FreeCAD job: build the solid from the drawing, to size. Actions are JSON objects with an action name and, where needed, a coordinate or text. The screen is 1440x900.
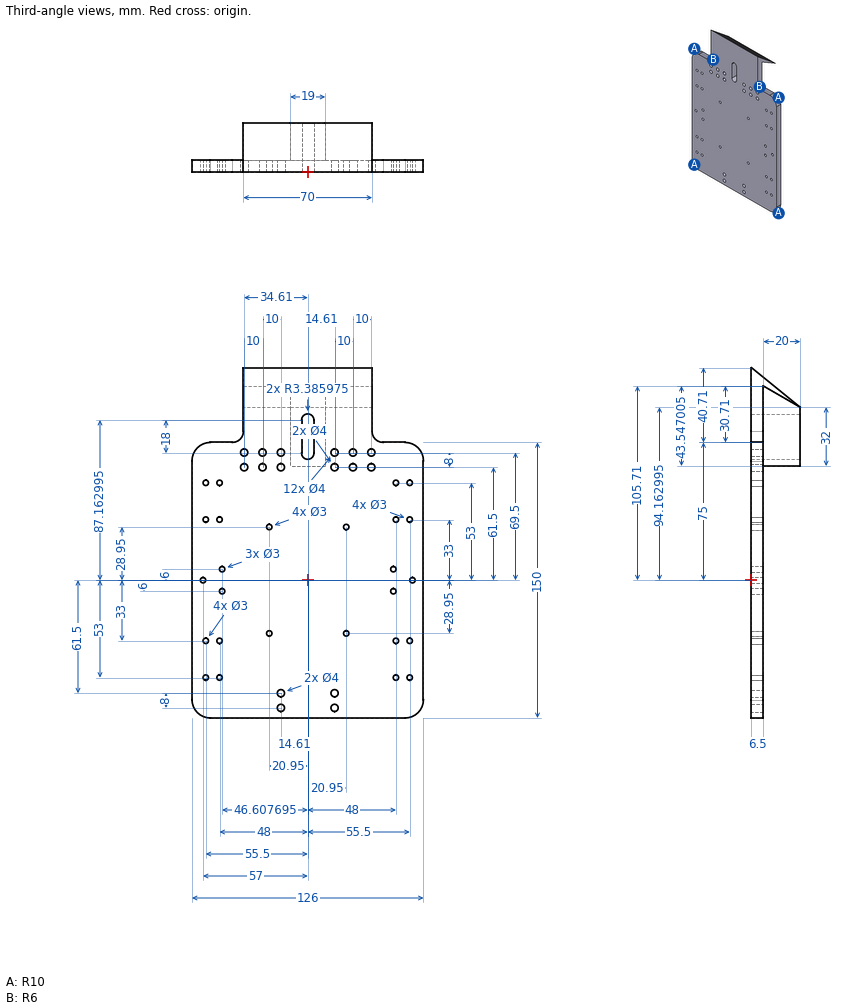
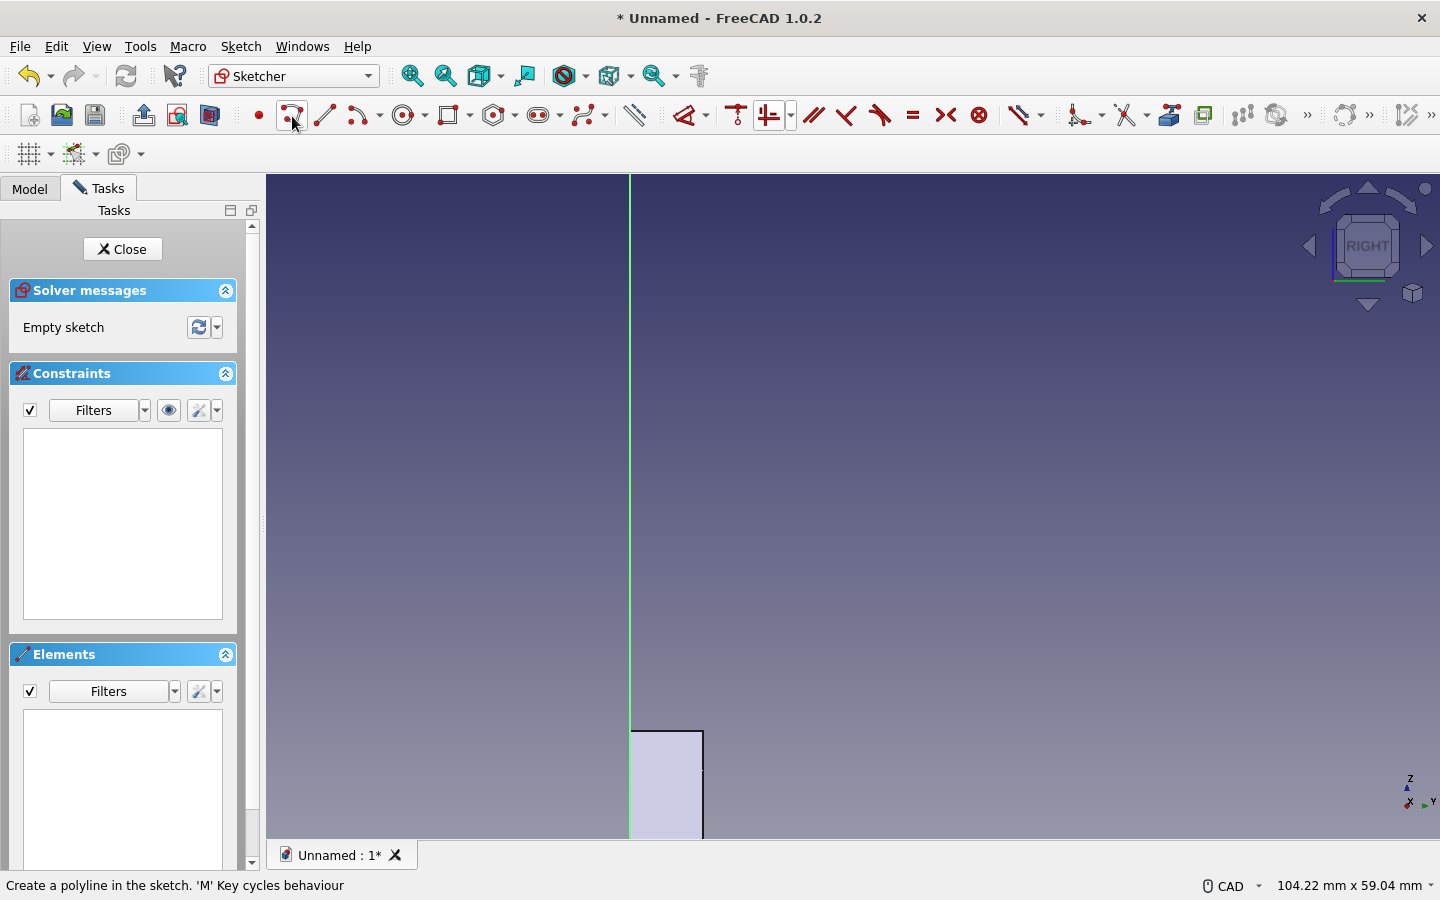
{"action": "left_click", "coordinate": [630, 731]}
{"action": "left_click", "coordinate": [703, 731]}
{"action": "left_click", "coordinate": [703, 385]}
{"action": "left_click", "coordinate": [929, 515]}
{"action": "left_click", "coordinate": [639, 272]}
{"action": "left_click", "coordinate": [630, 732]}
{"action": "key", "text": "Escape"}
{"action": "key", "text": "Escape"}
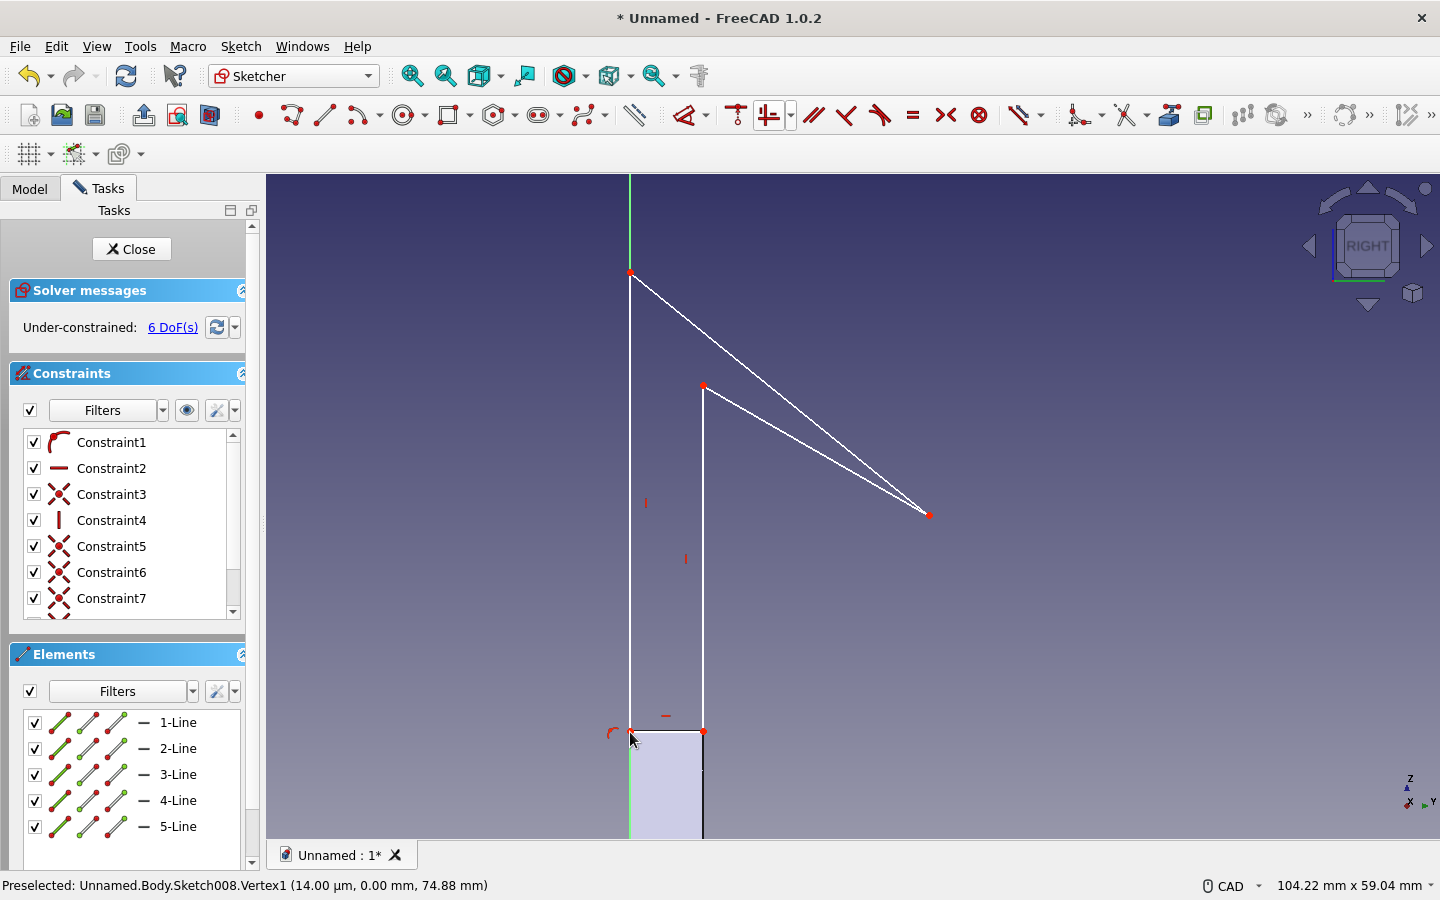
{"action": "left_click", "coordinate": [684, 116]}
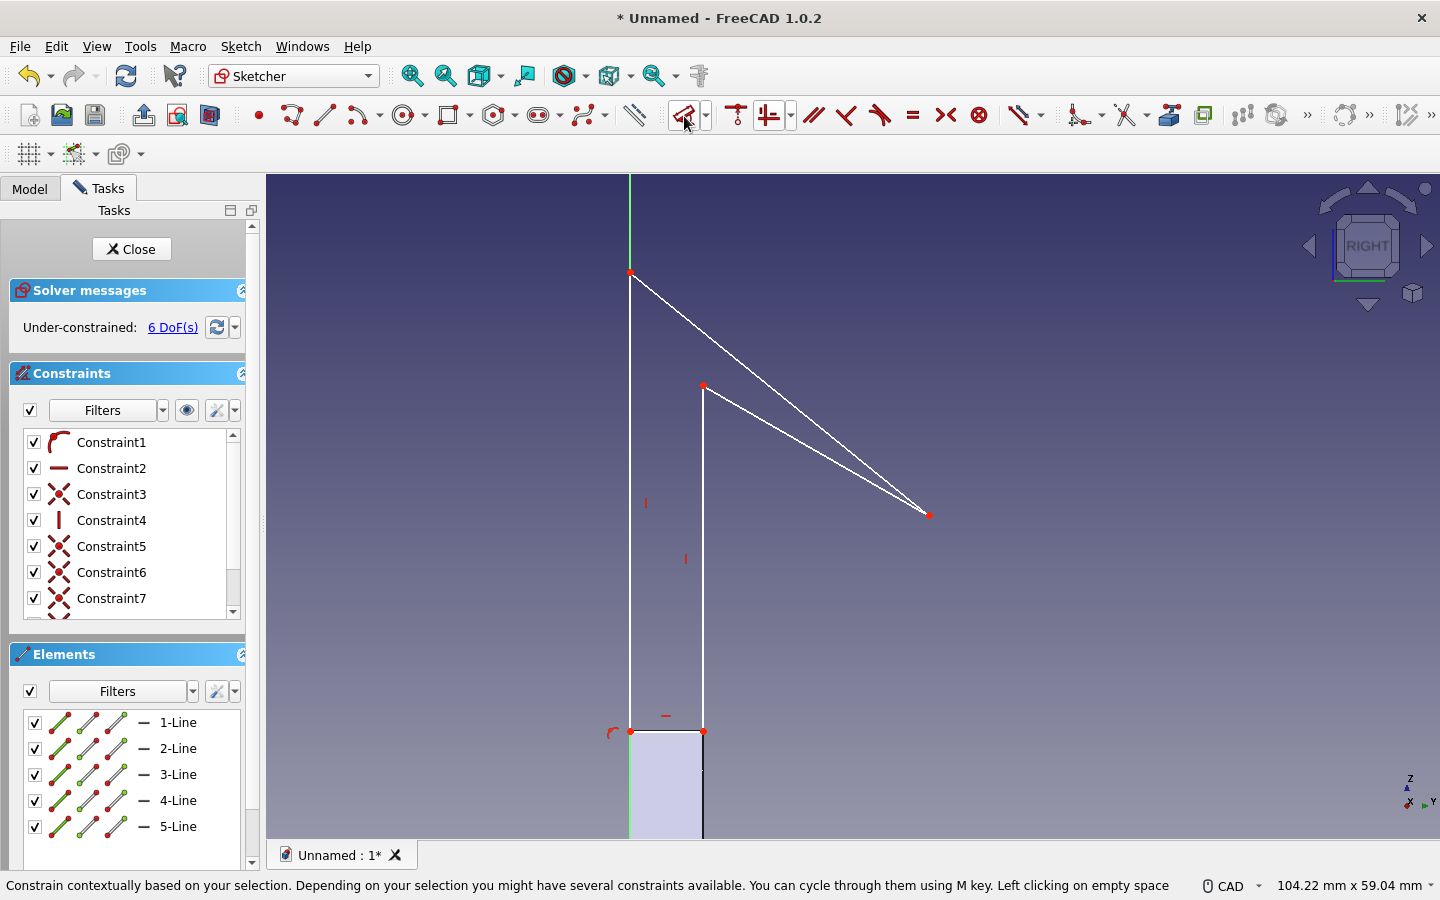
{"action": "left_click", "coordinate": [652, 732]}
{"action": "left_click", "coordinate": [667, 766]}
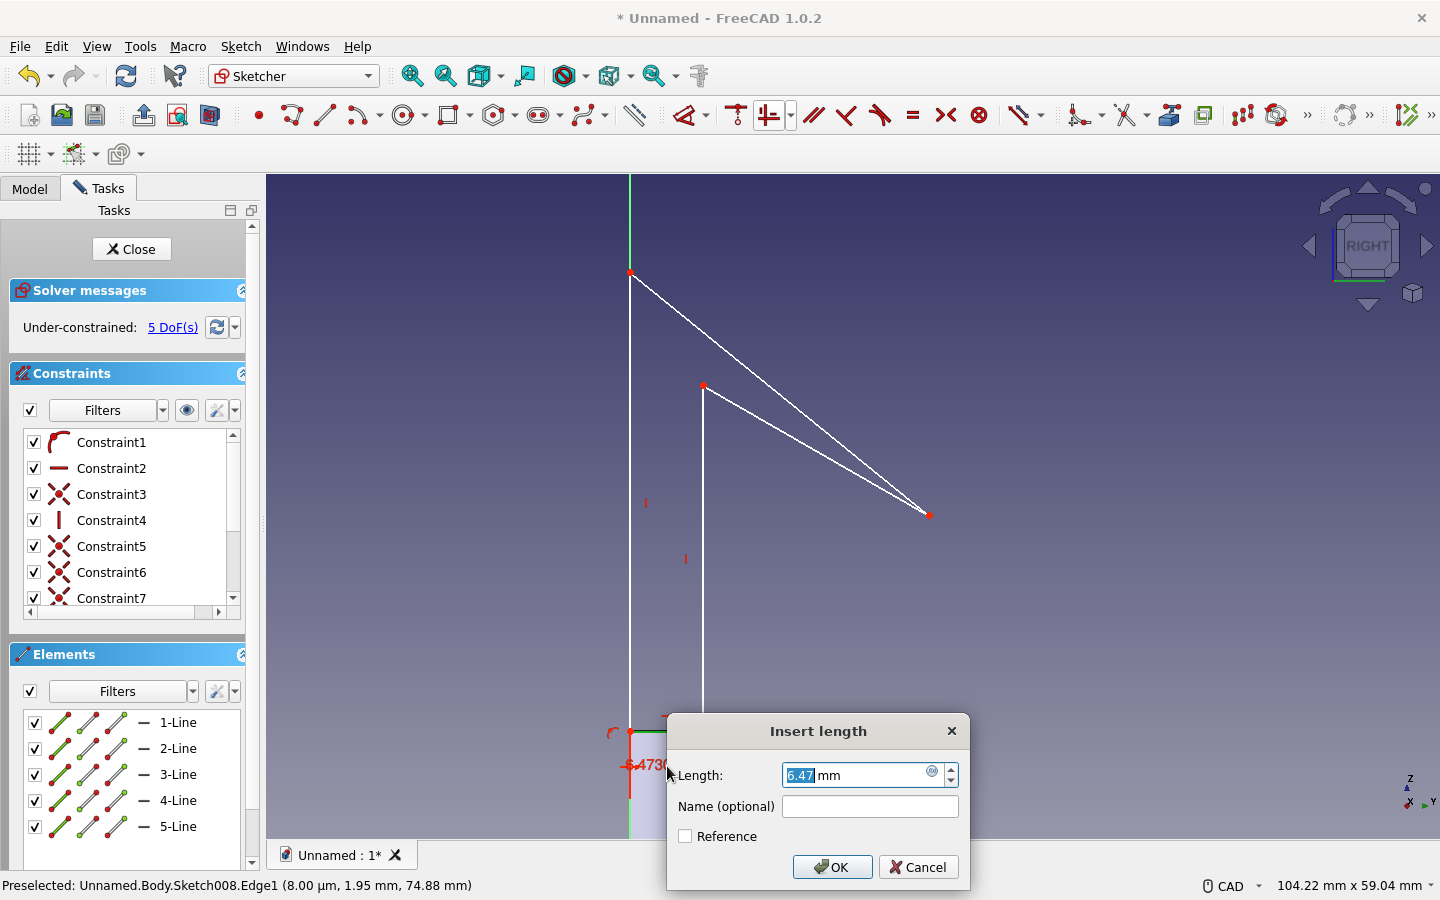
{"action": "type", "text": "6.5"}
{"action": "key", "text": "Return"}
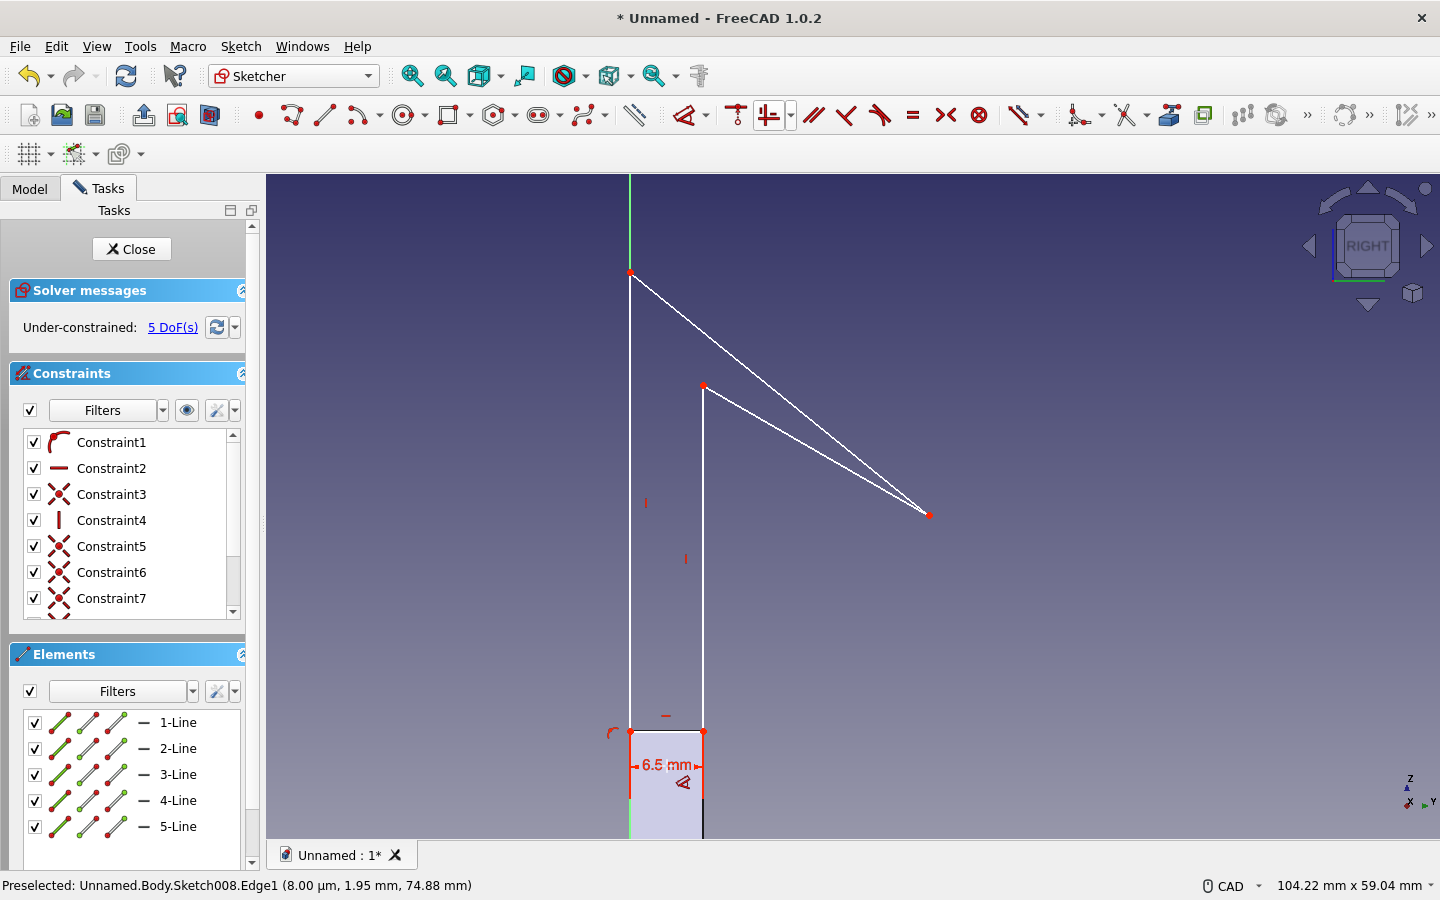
{"action": "left_click", "coordinate": [630, 732]}
{"action": "left_click", "coordinate": [596, 772]}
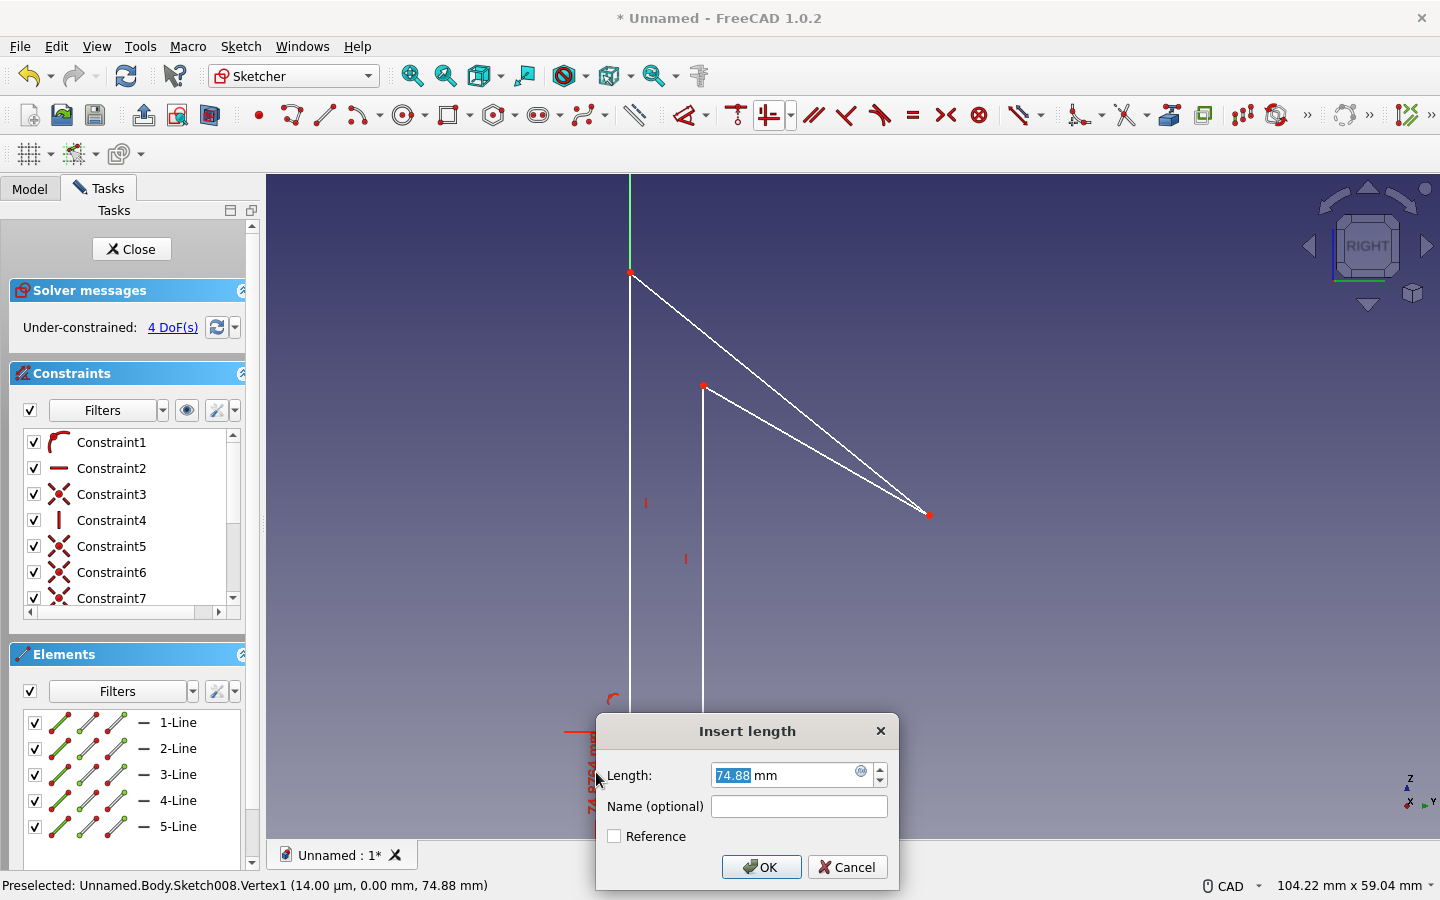
{"action": "type", "text": "75"}
{"action": "key", "text": "Return"}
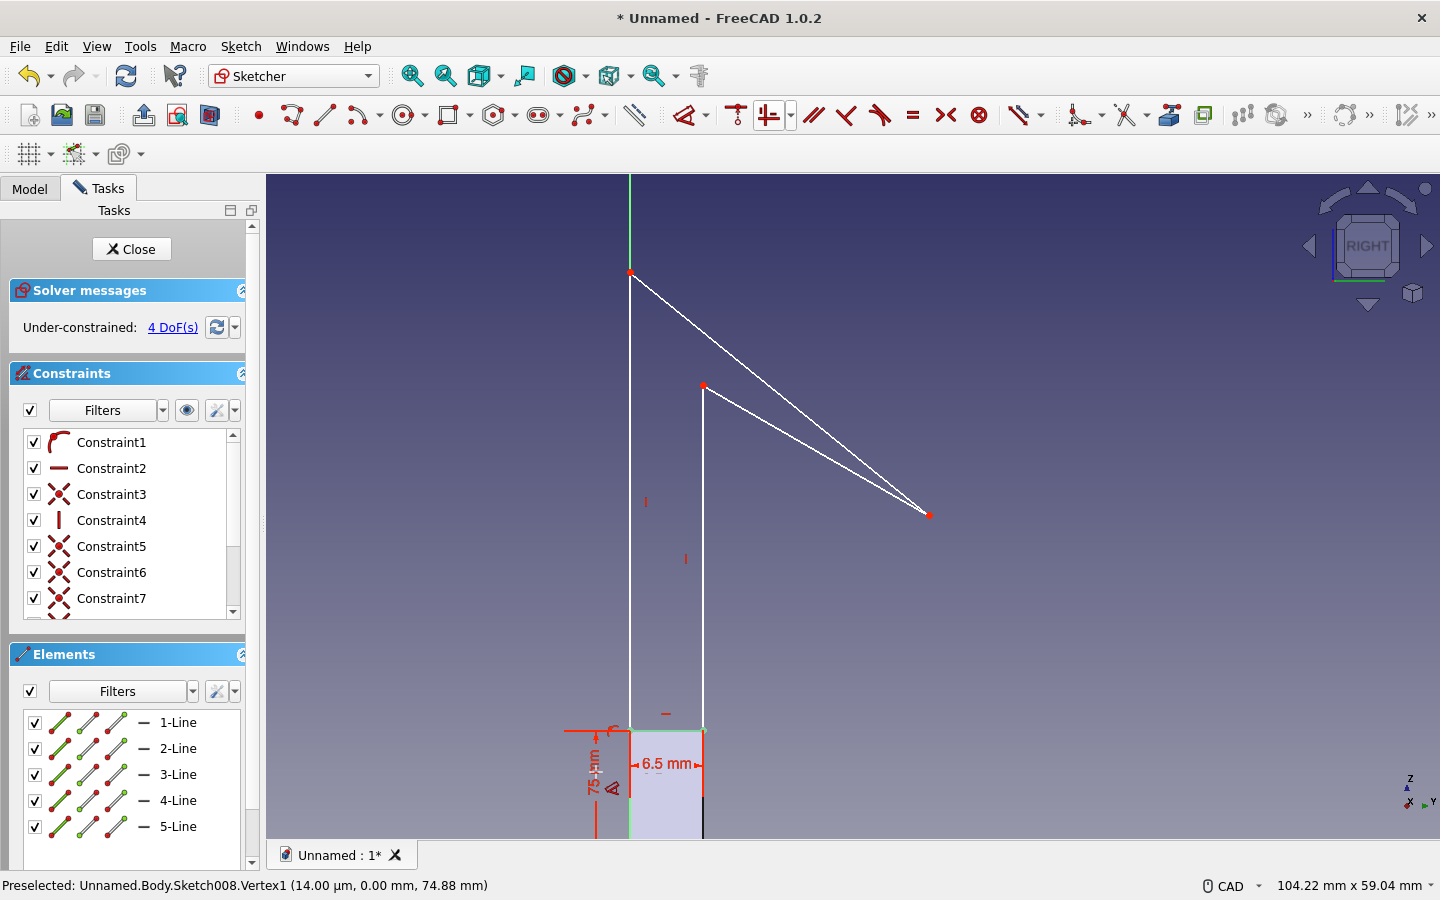
{"action": "left_click", "coordinate": [771, 425]}
{"action": "left_click", "coordinate": [816, 352]}